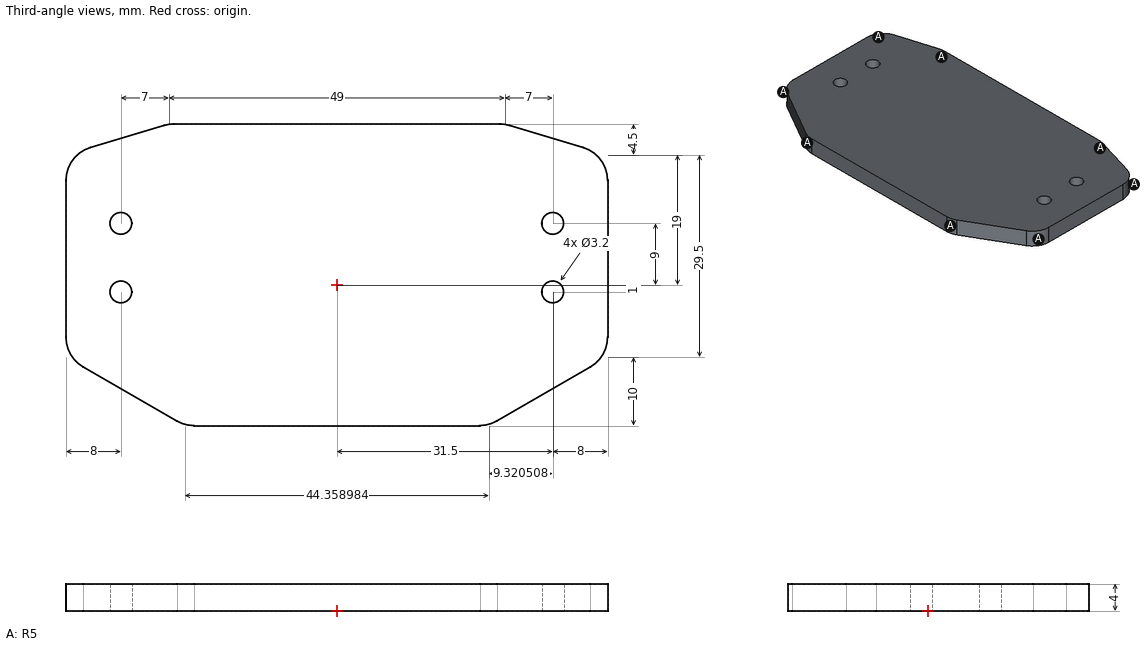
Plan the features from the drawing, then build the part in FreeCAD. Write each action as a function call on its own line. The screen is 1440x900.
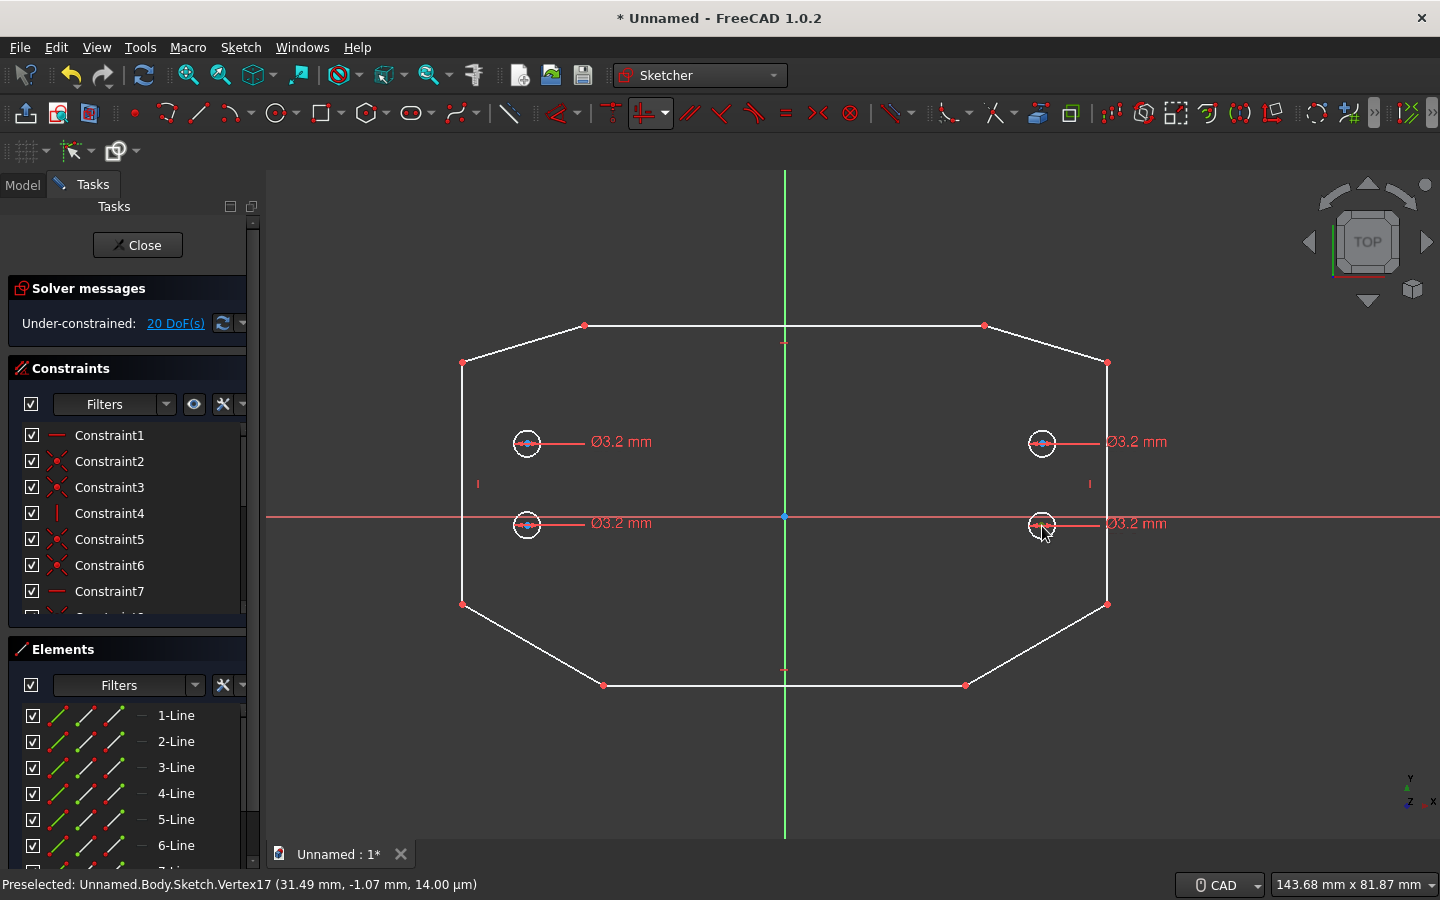
click(1042, 444)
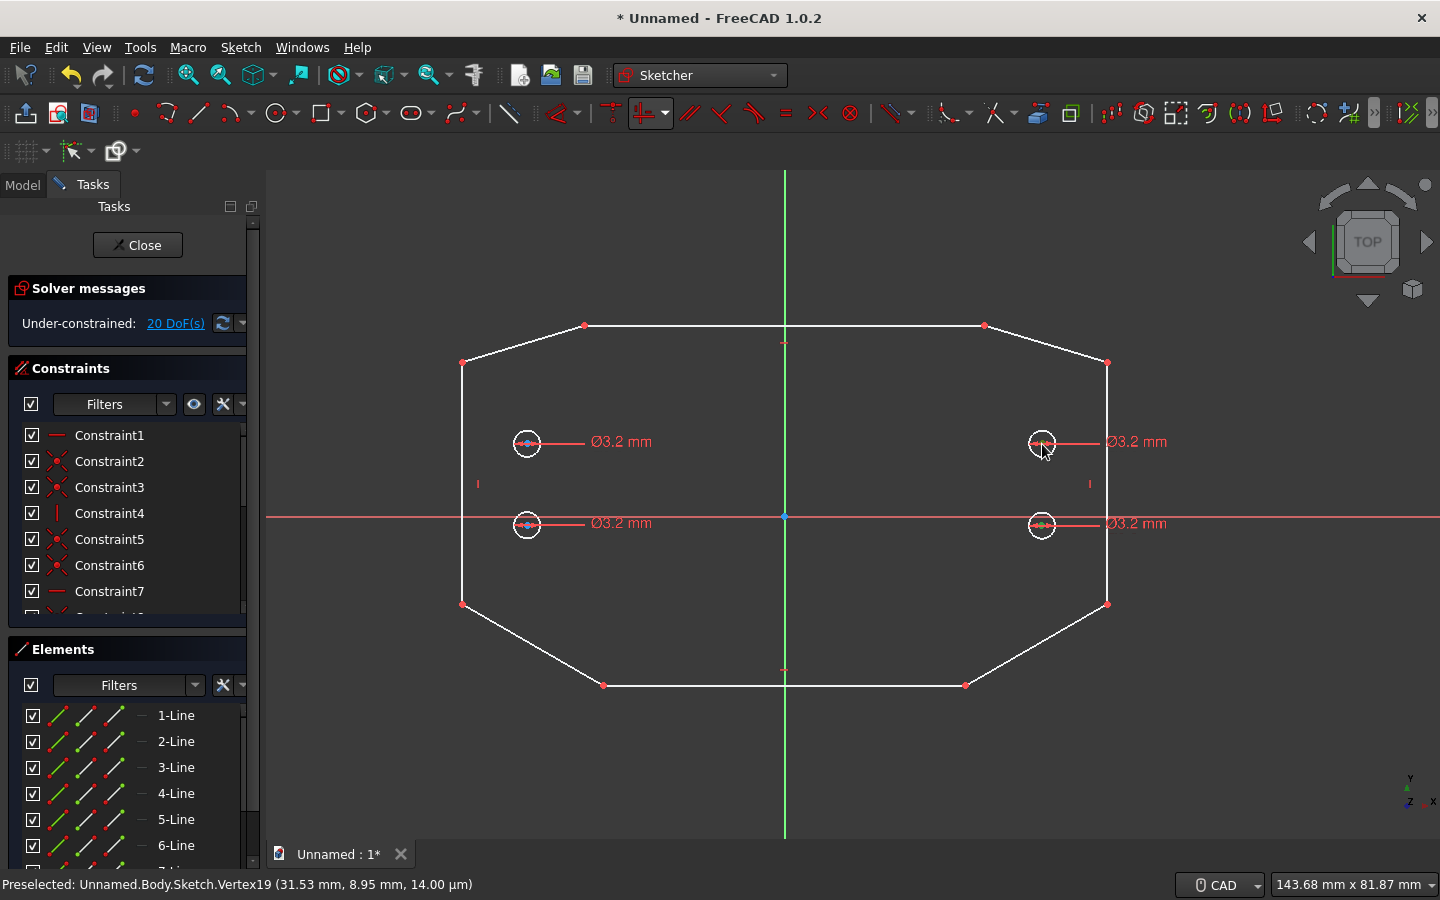
click(668, 114)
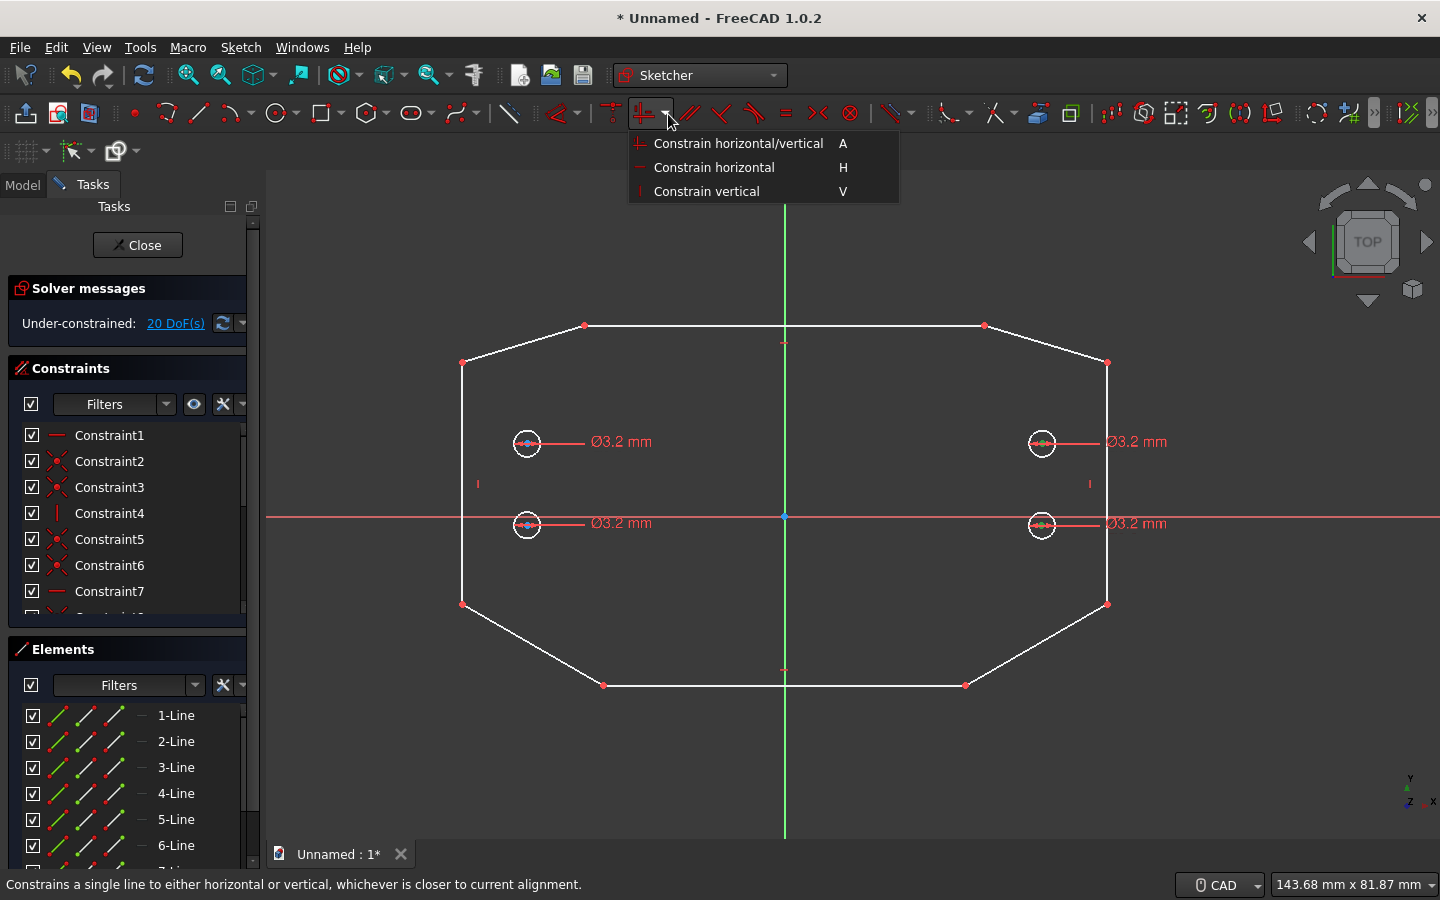
click(764, 191)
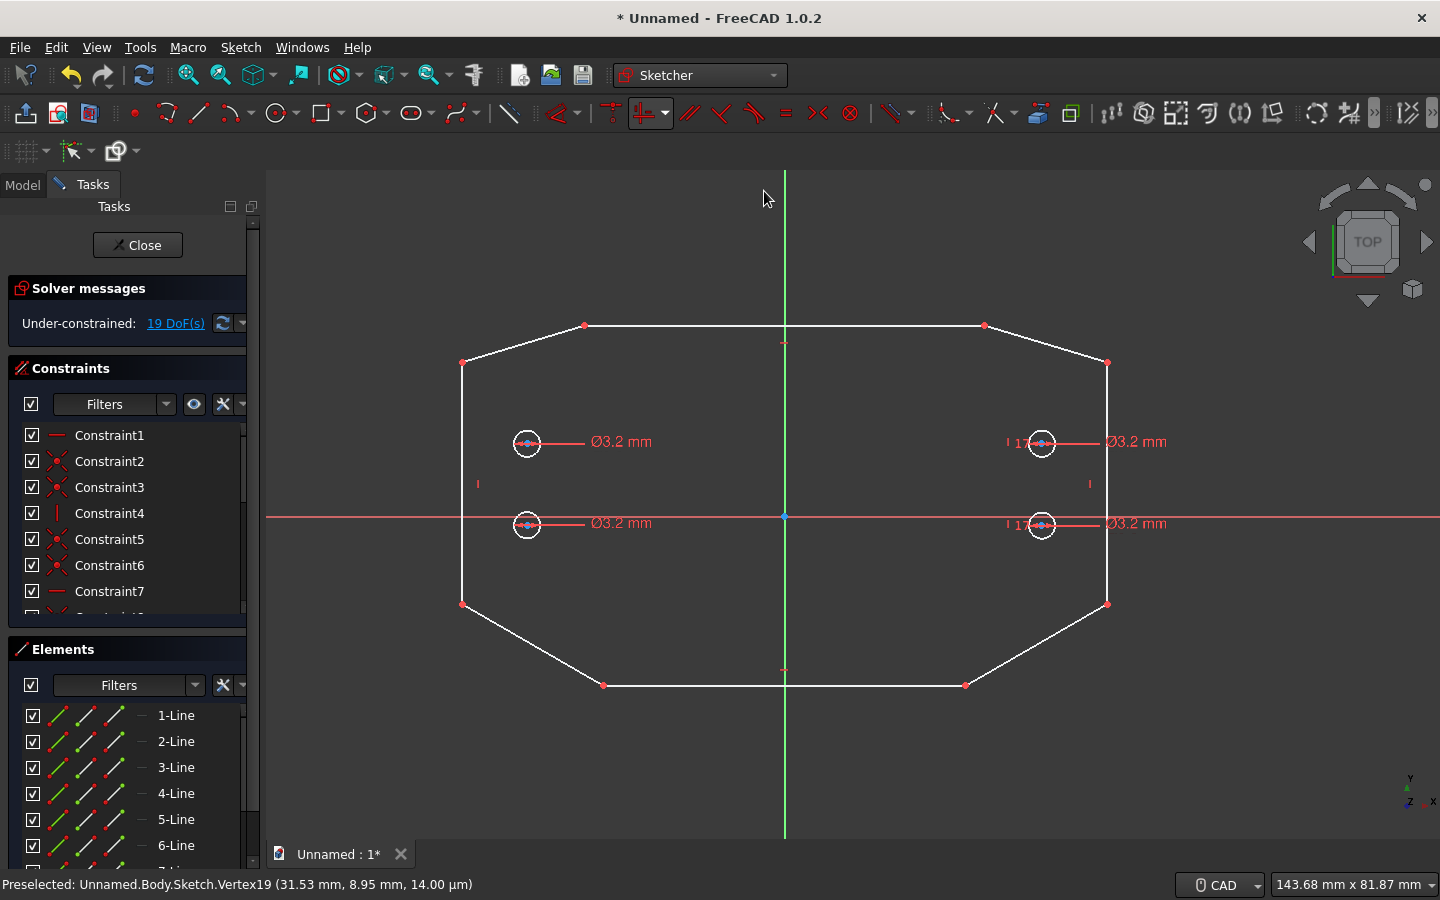
click(527, 525)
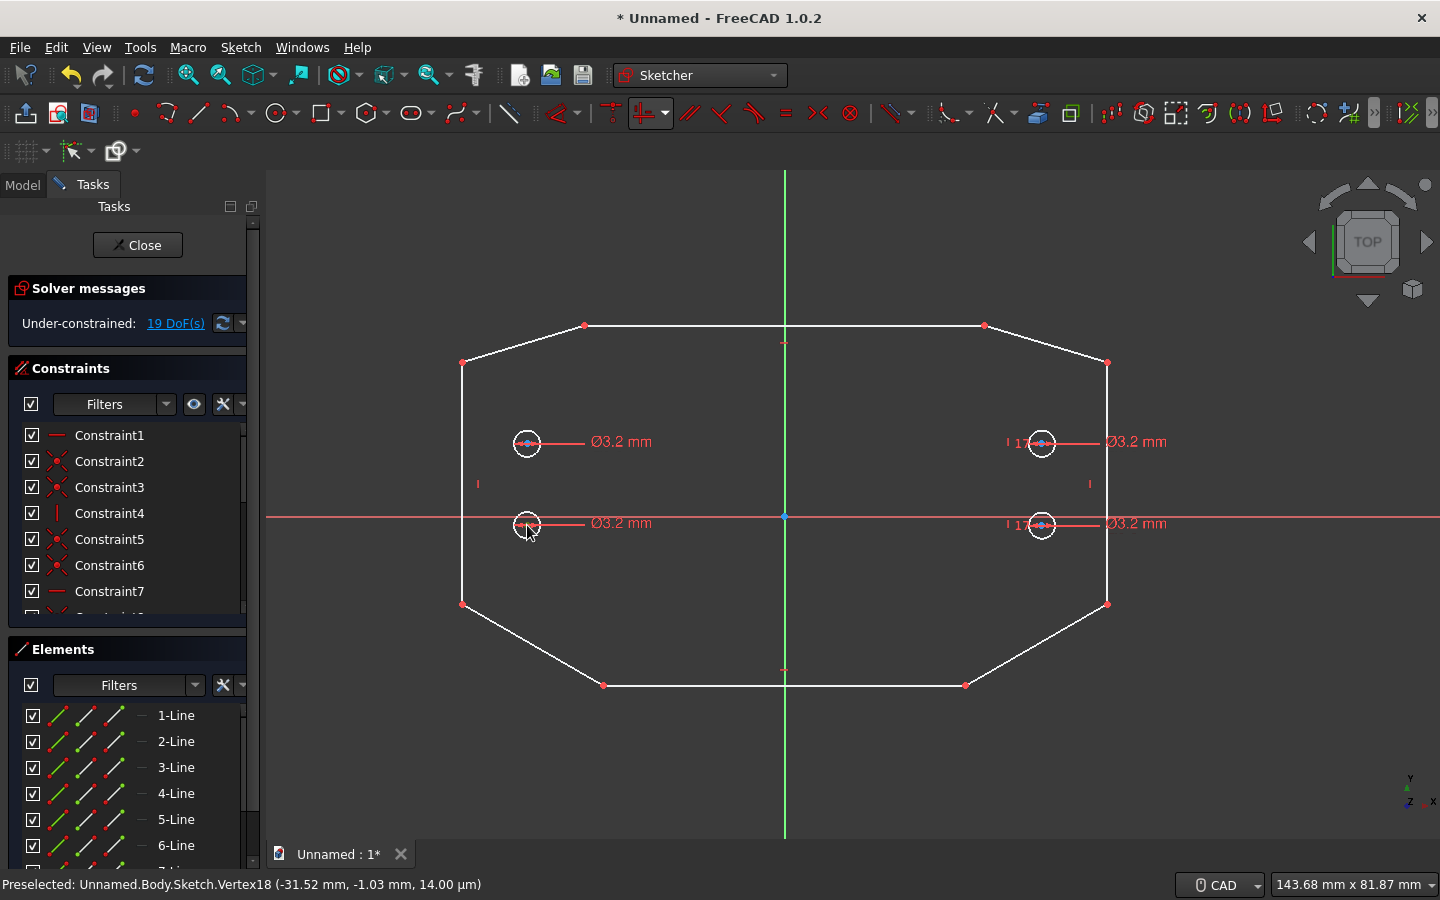
click(527, 444)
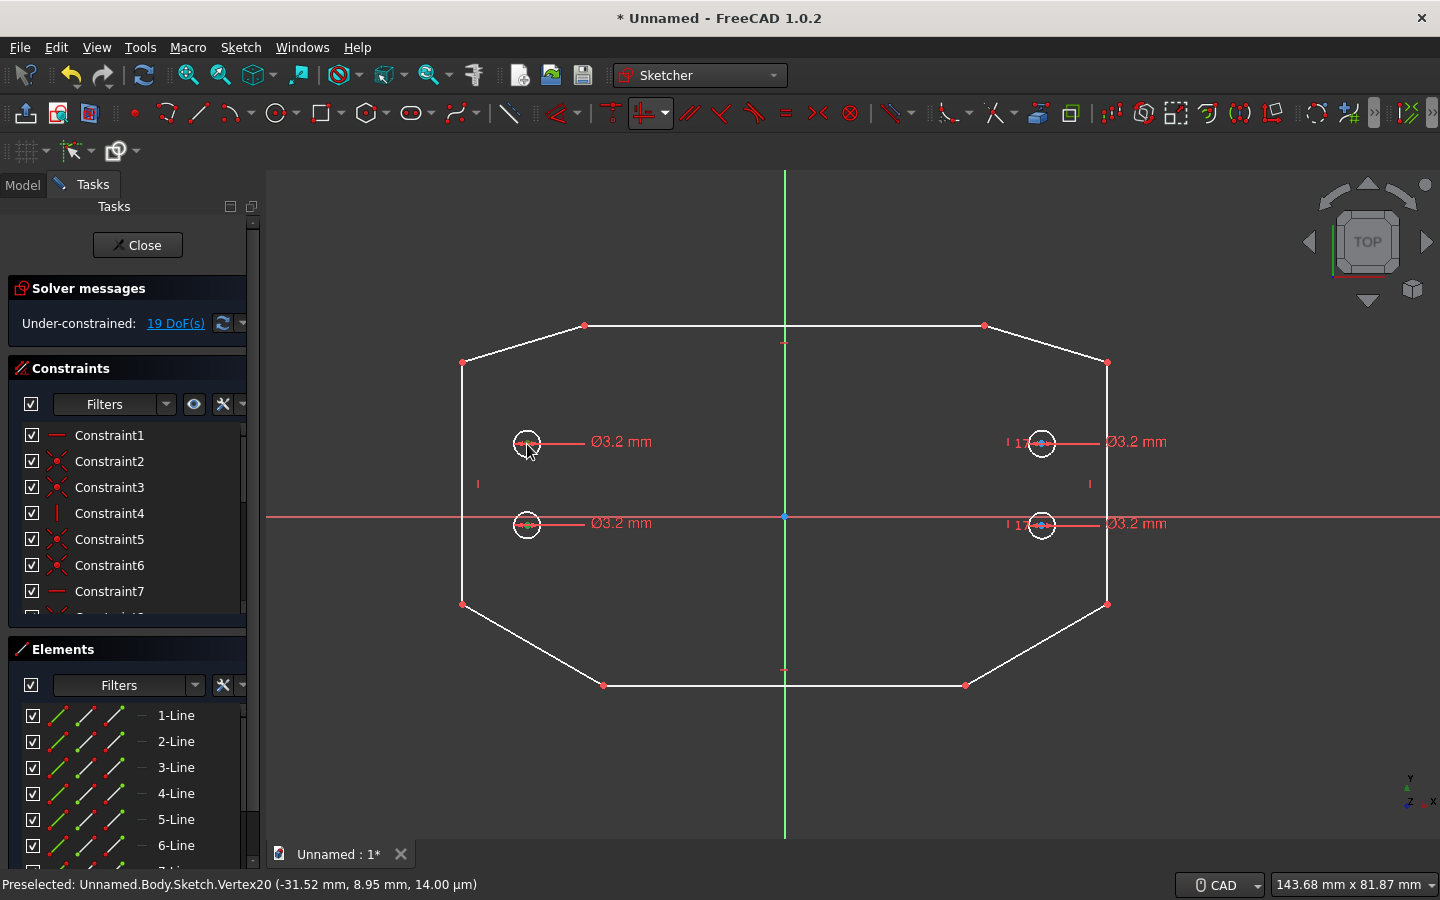
key(v)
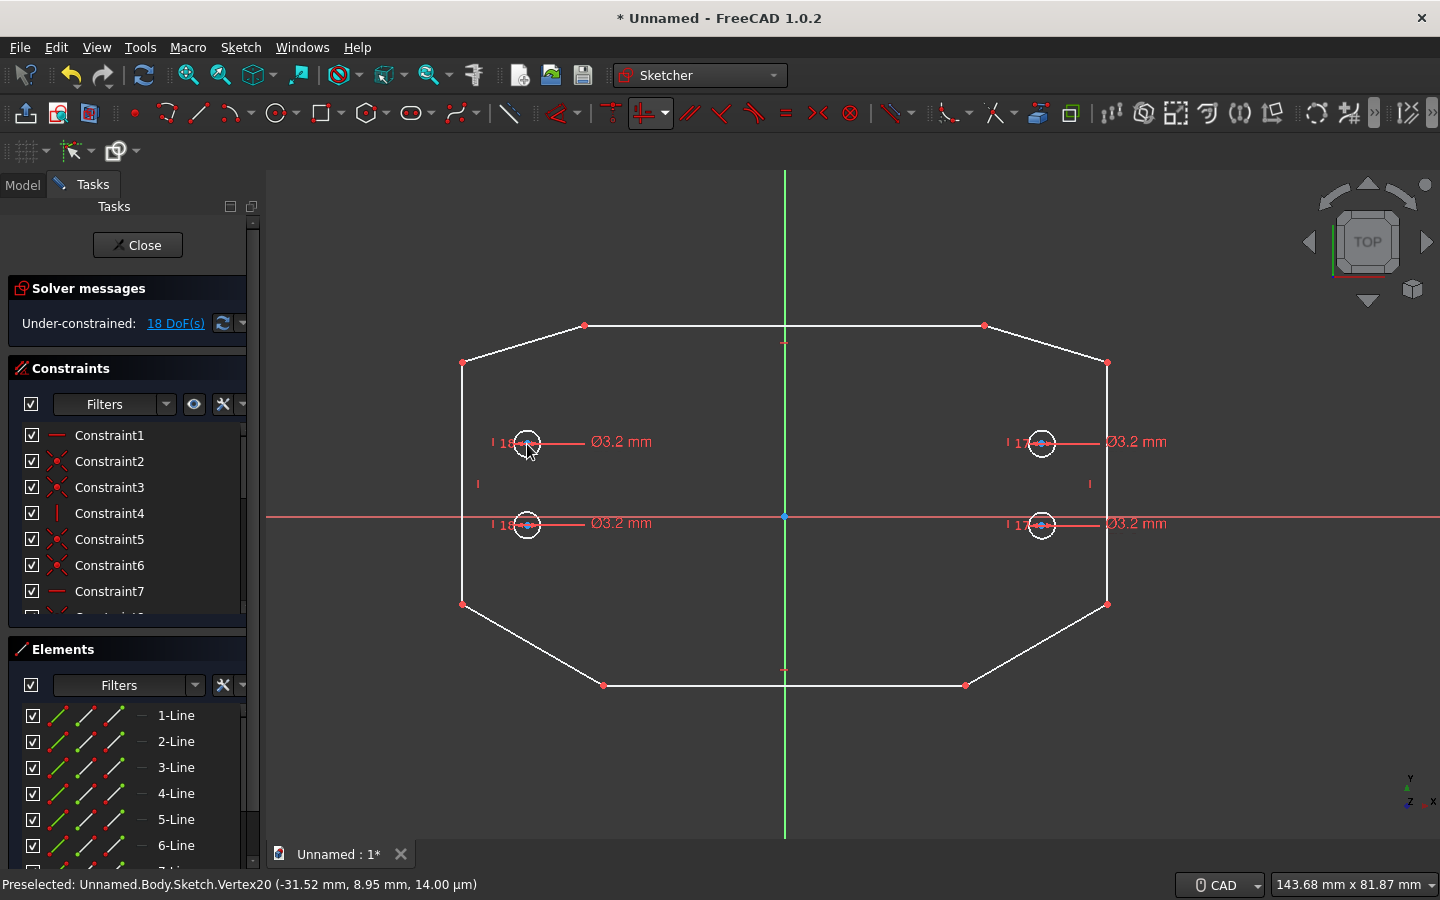
click(556, 114)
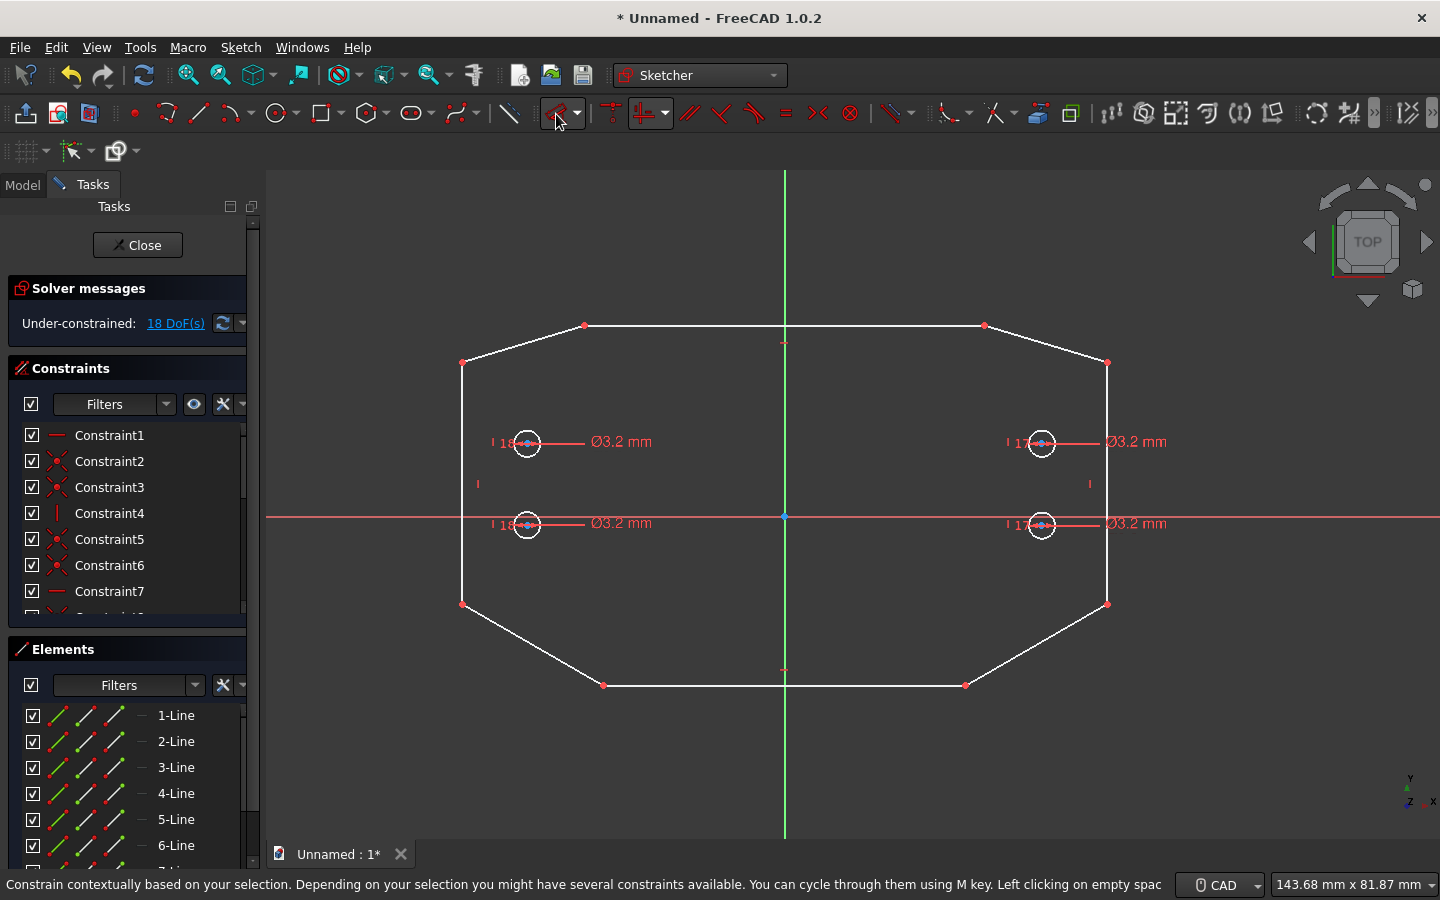
scroll(1042, 526, up, 8)